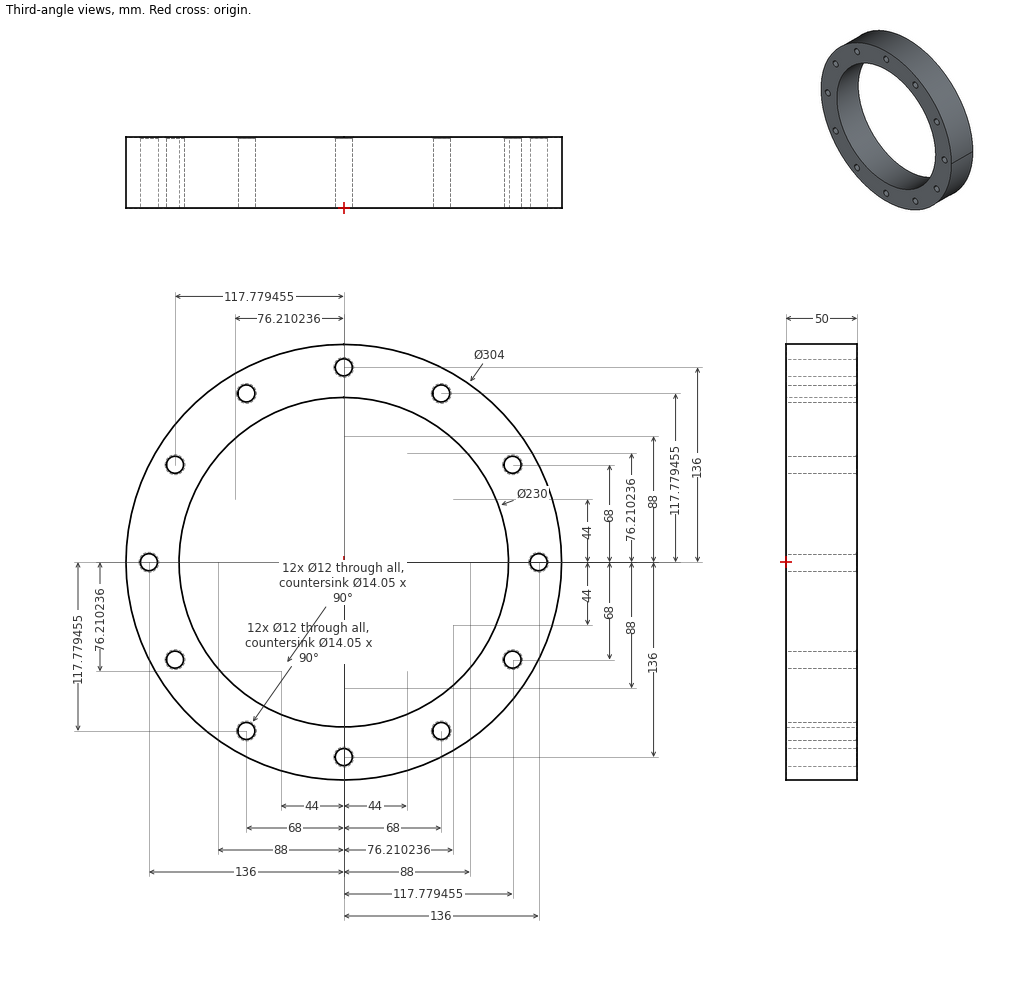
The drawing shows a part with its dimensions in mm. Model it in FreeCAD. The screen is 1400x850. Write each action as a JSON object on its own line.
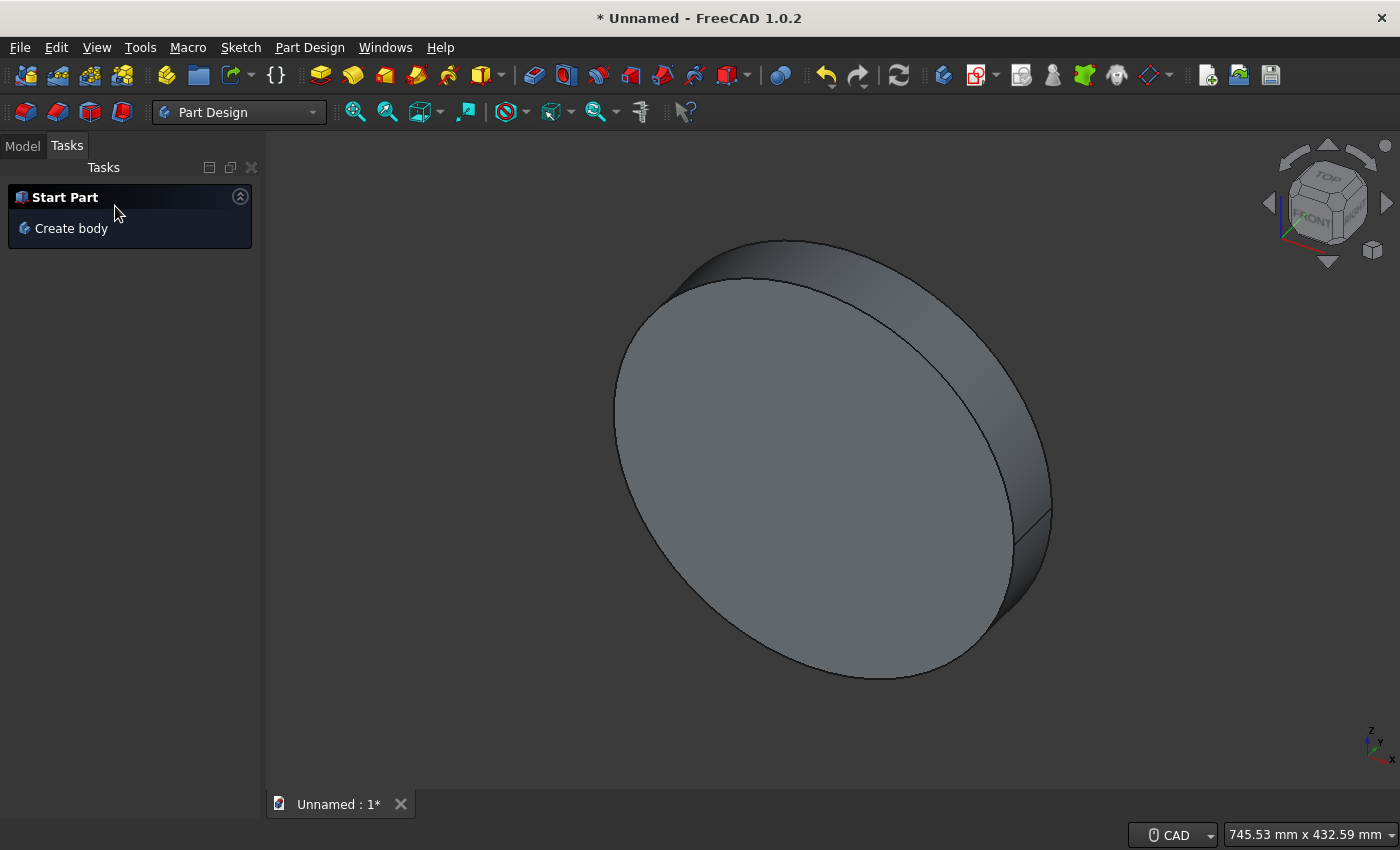
{"action": "key", "text": "4"}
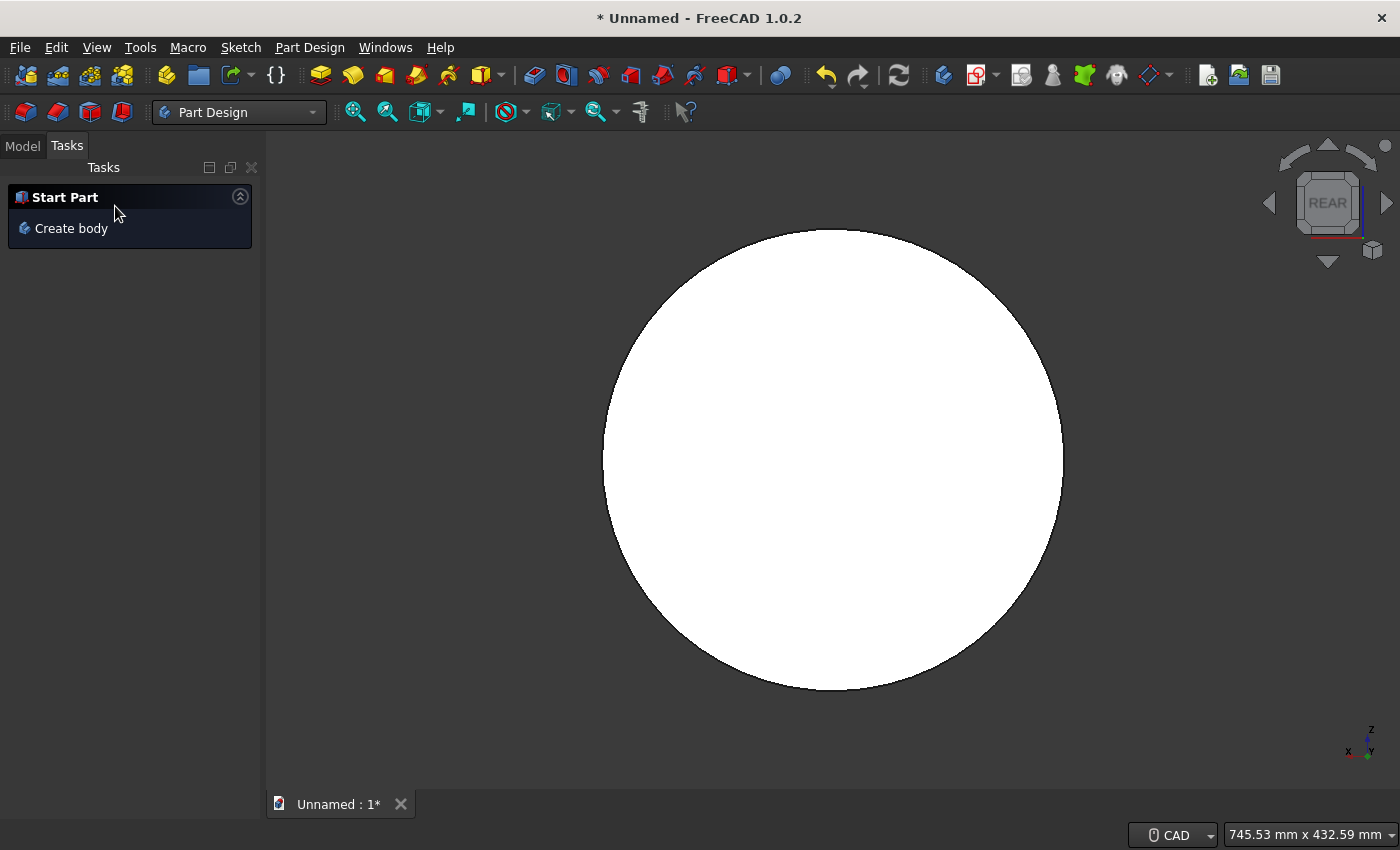
{"action": "left_click", "coordinate": [833, 459]}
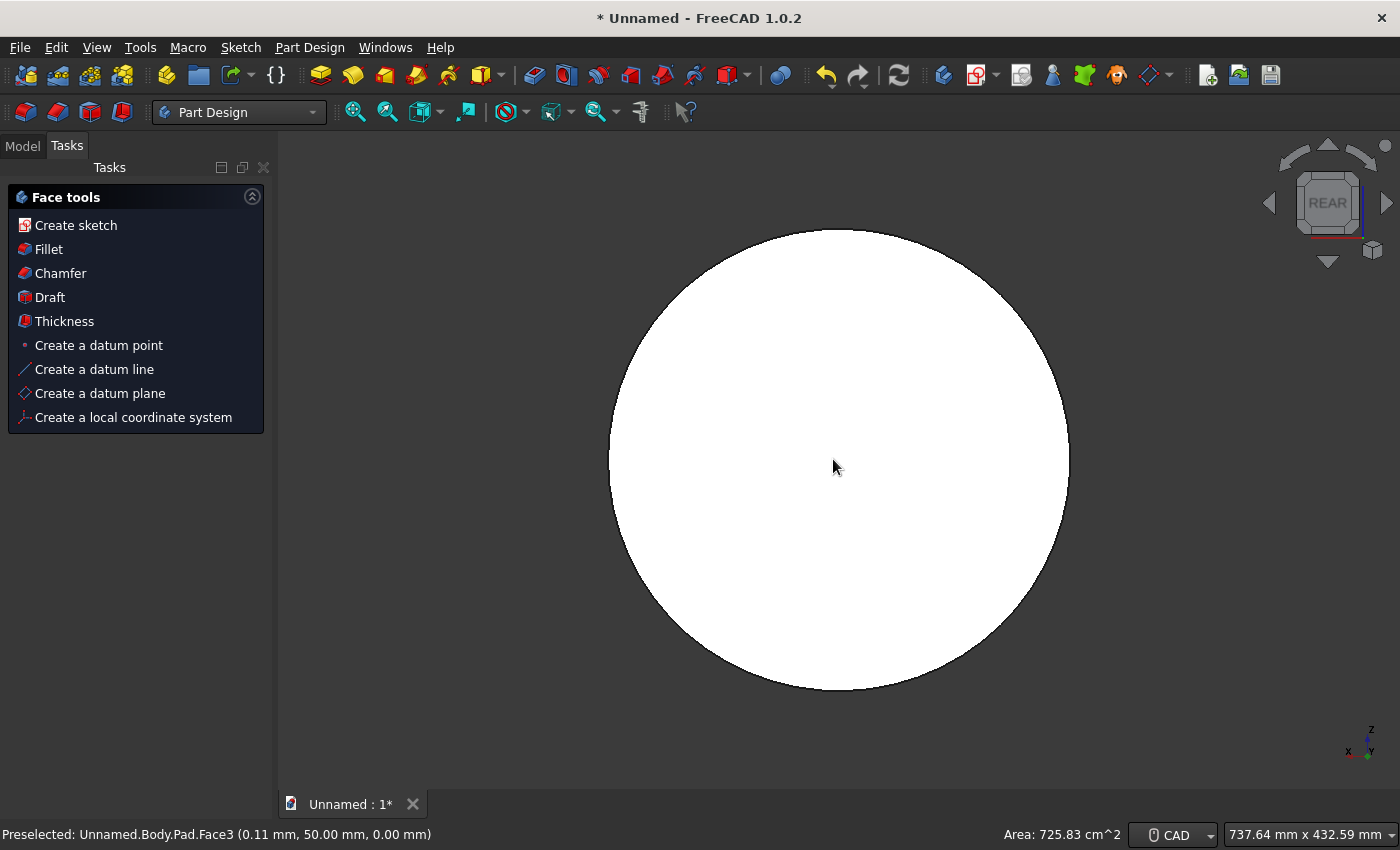
{"action": "left_click", "coordinate": [976, 76]}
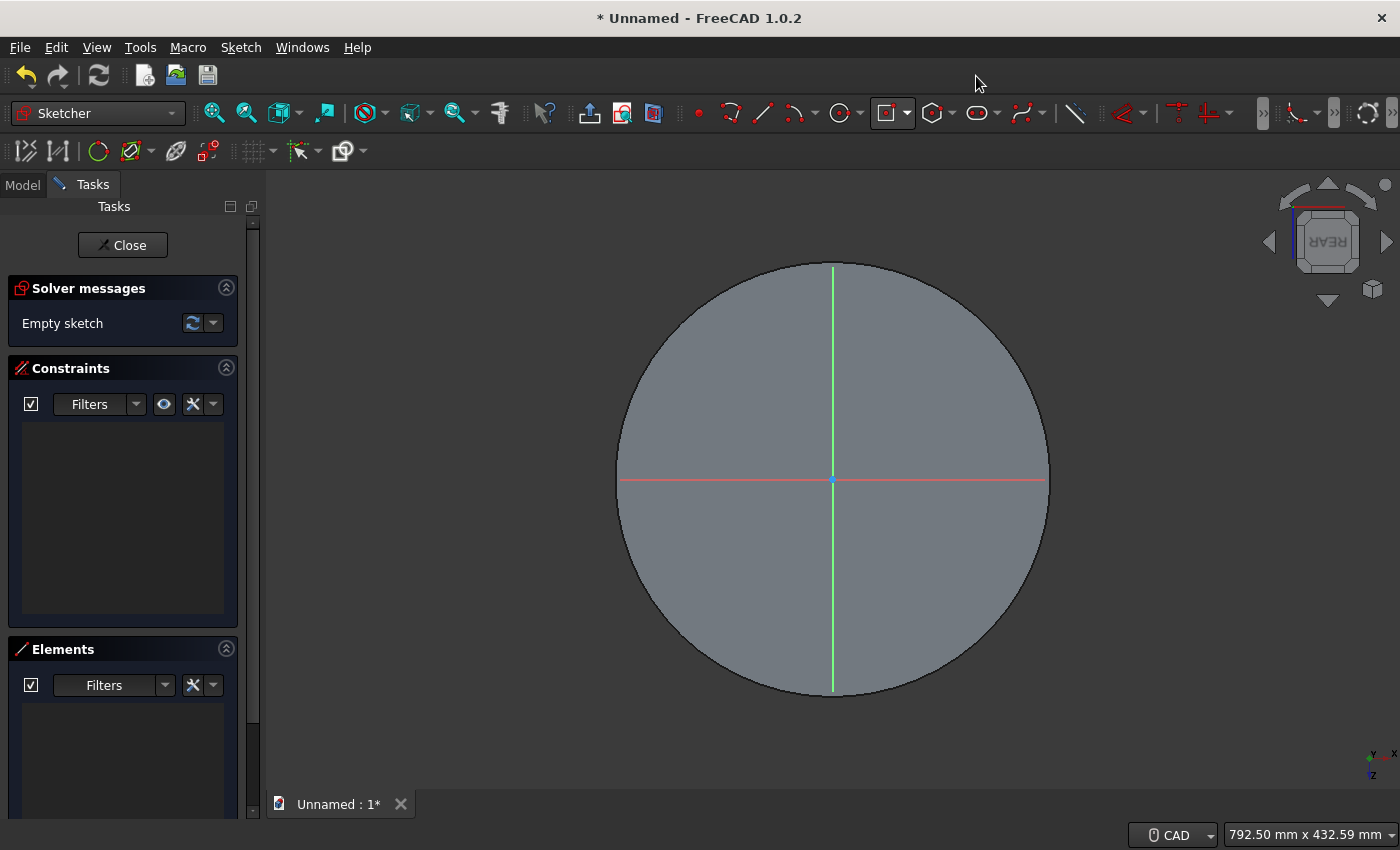
{"action": "key", "text": "g c"}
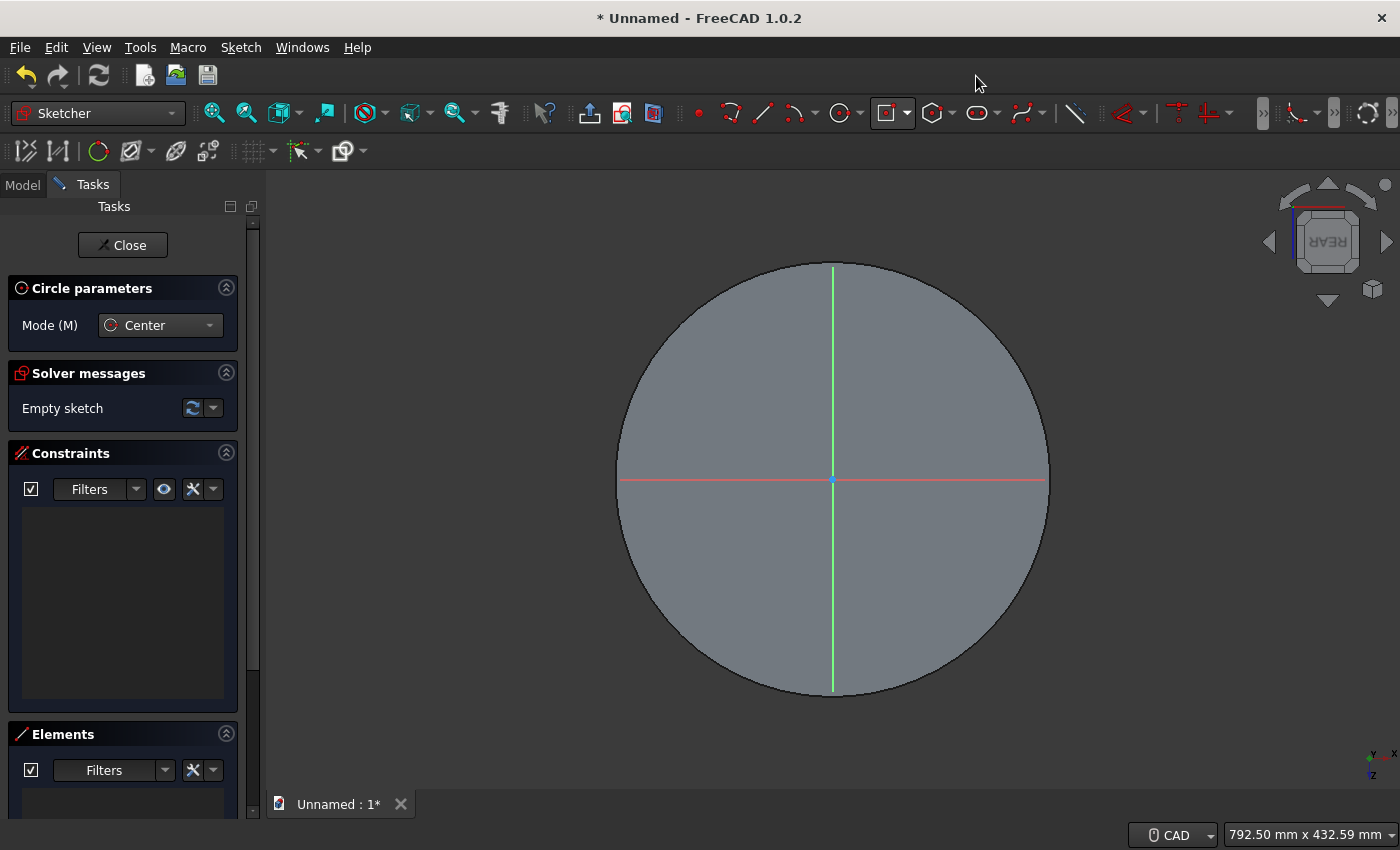
{"action": "scroll", "coordinate": [736, 311], "scroll_direction": "up", "scroll_amount": 5}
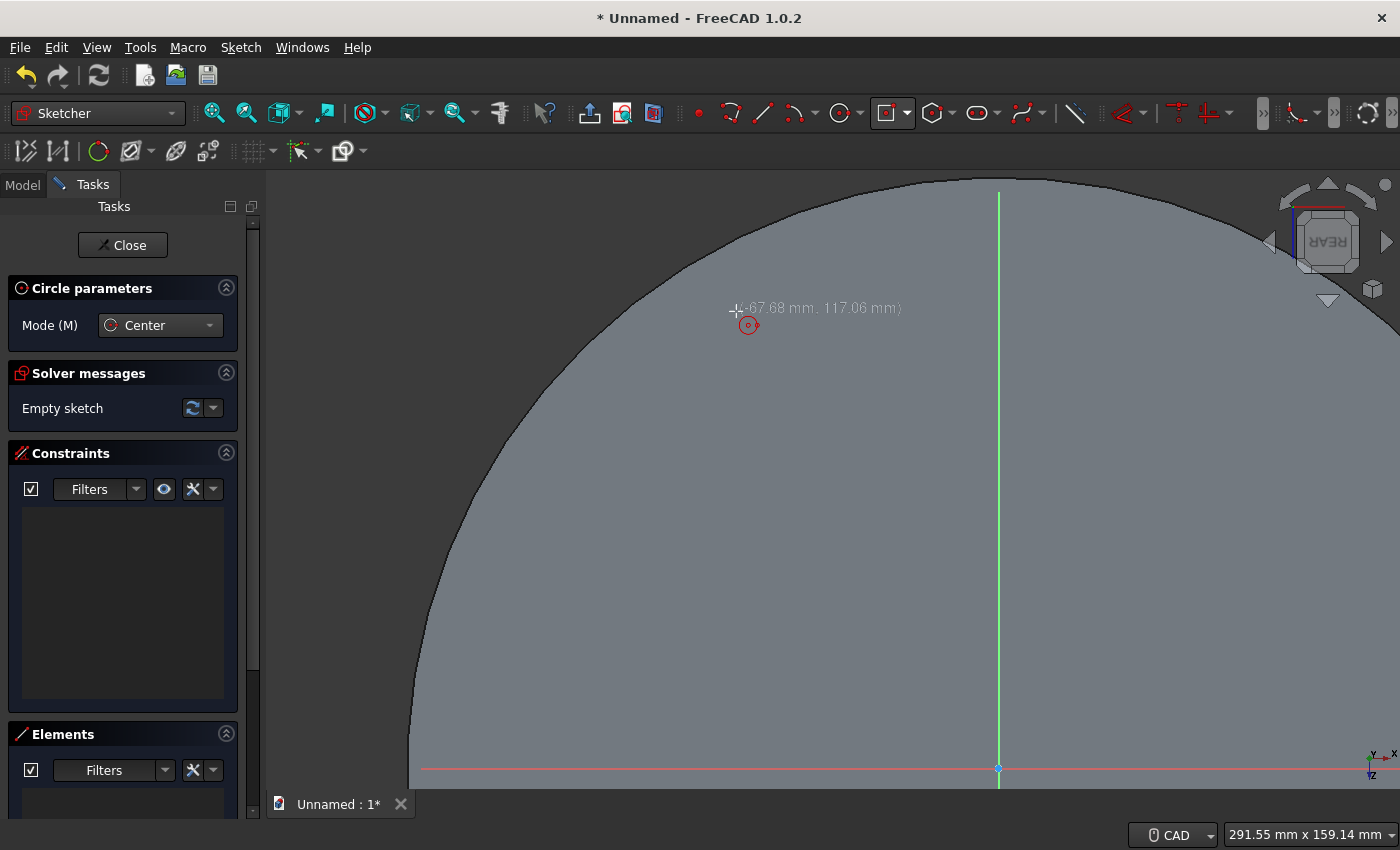
{"action": "left_click", "coordinate": [734, 311]}
{"action": "left_click", "coordinate": [751, 294]}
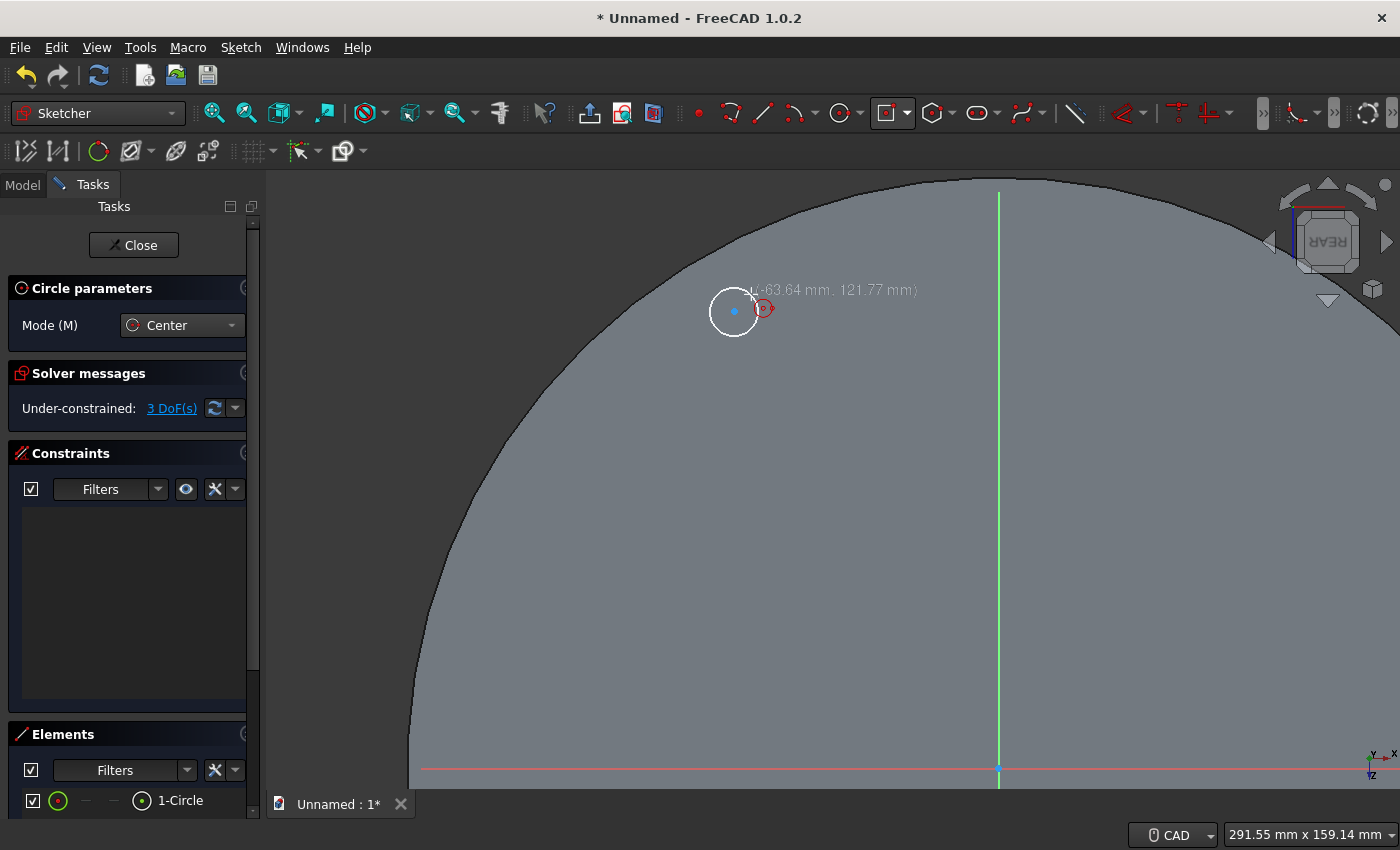
{"action": "left_click", "coordinate": [999, 240]}
{"action": "left_click", "coordinate": [1015, 223]}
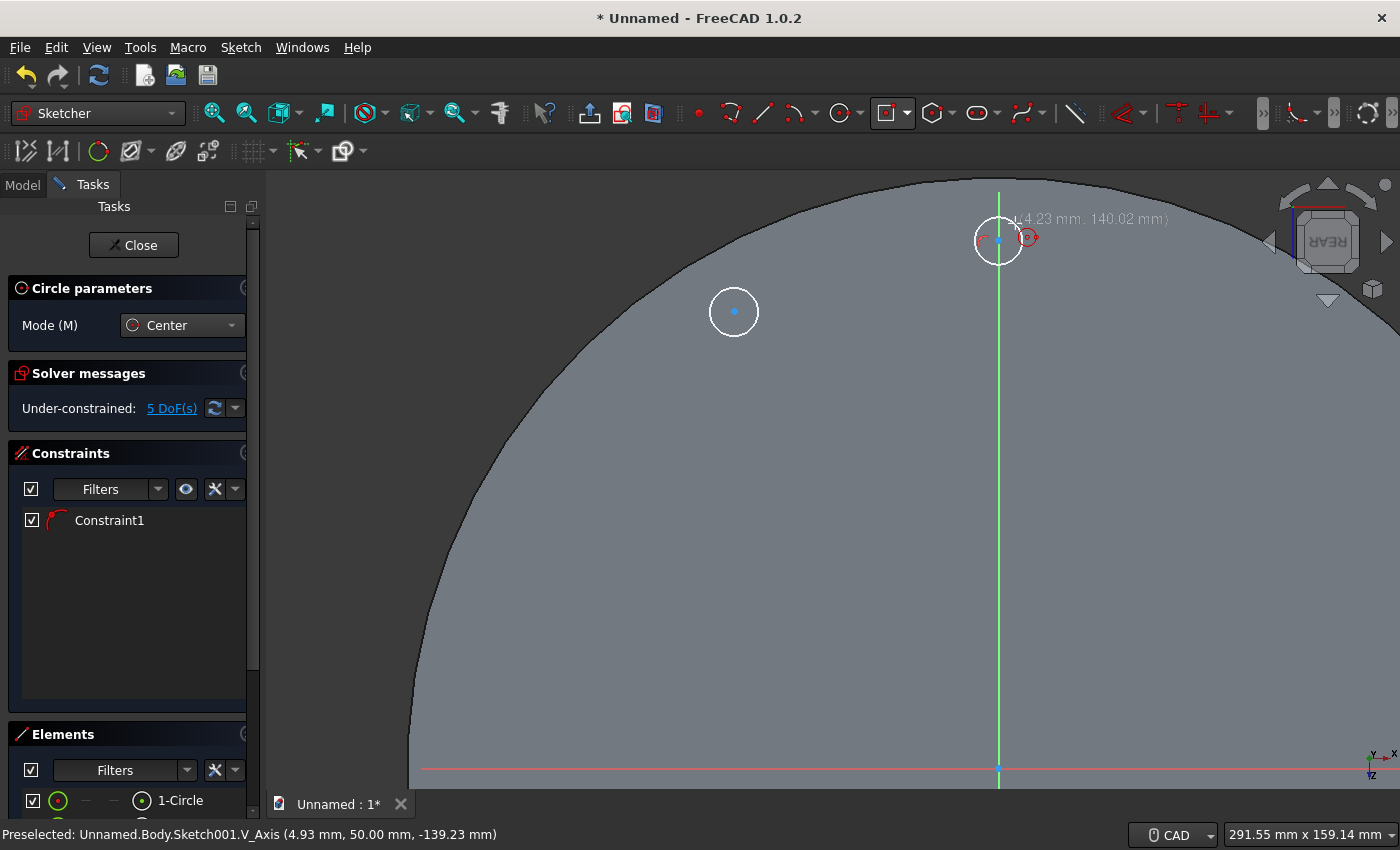
{"action": "scroll", "coordinate": [628, 311], "scroll_direction": "down", "scroll_amount": 5}